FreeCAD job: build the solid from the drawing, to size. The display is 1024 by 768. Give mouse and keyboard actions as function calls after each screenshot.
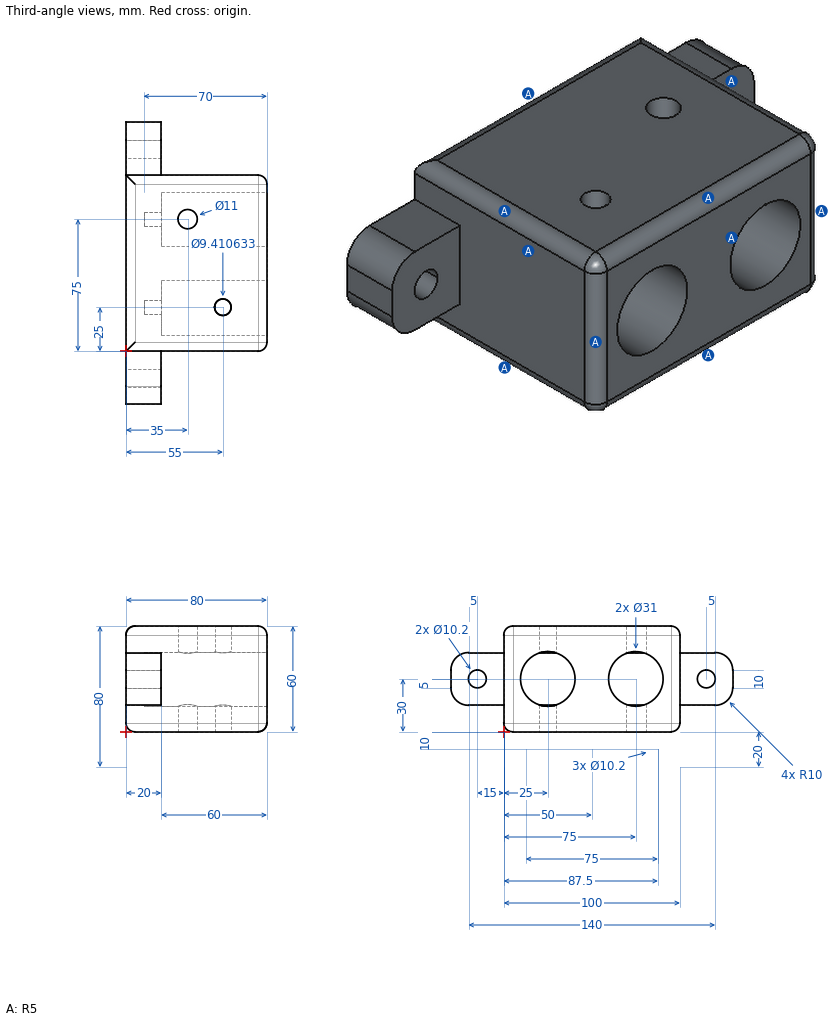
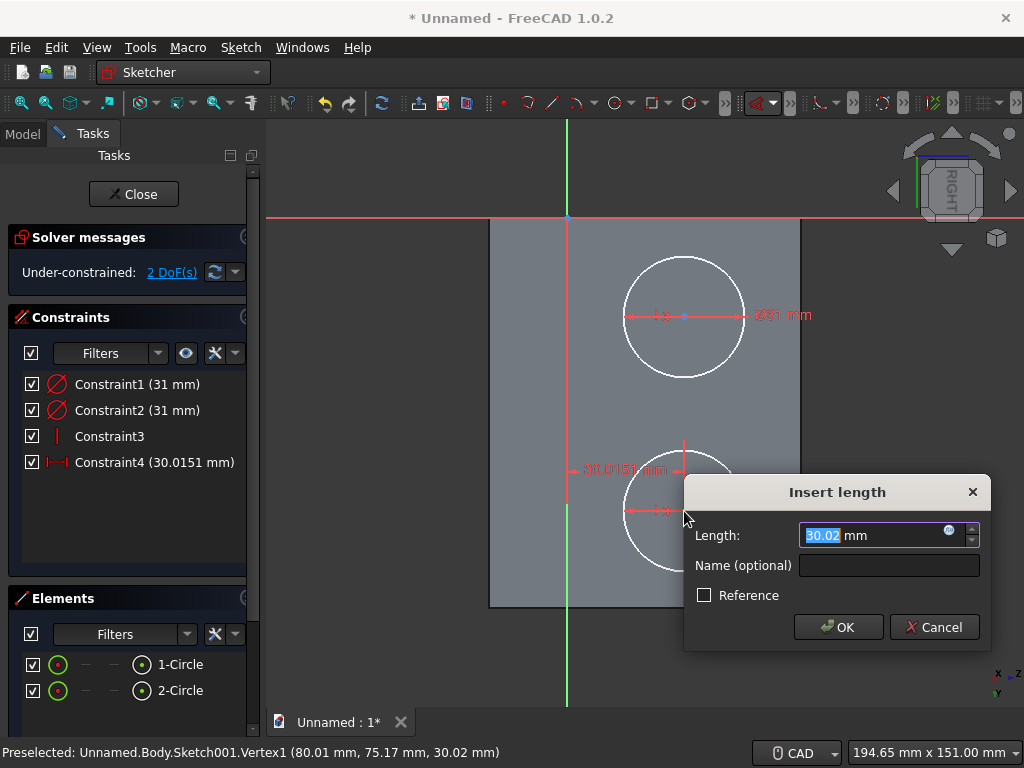
text(30)
key(Return)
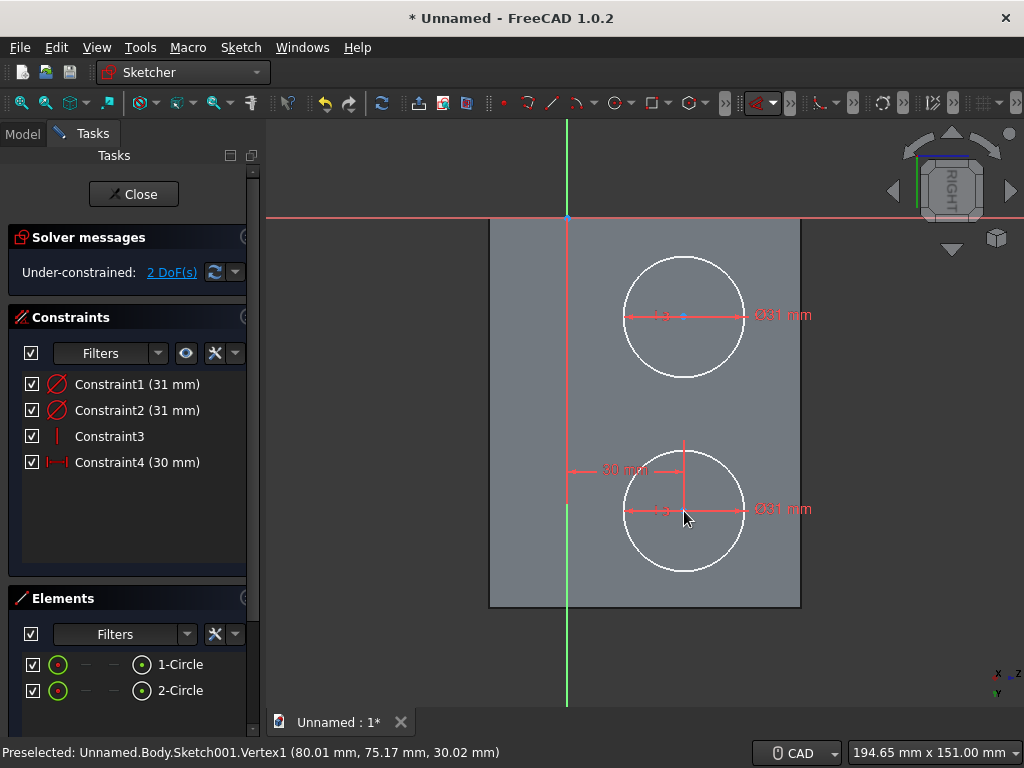
click(684, 511)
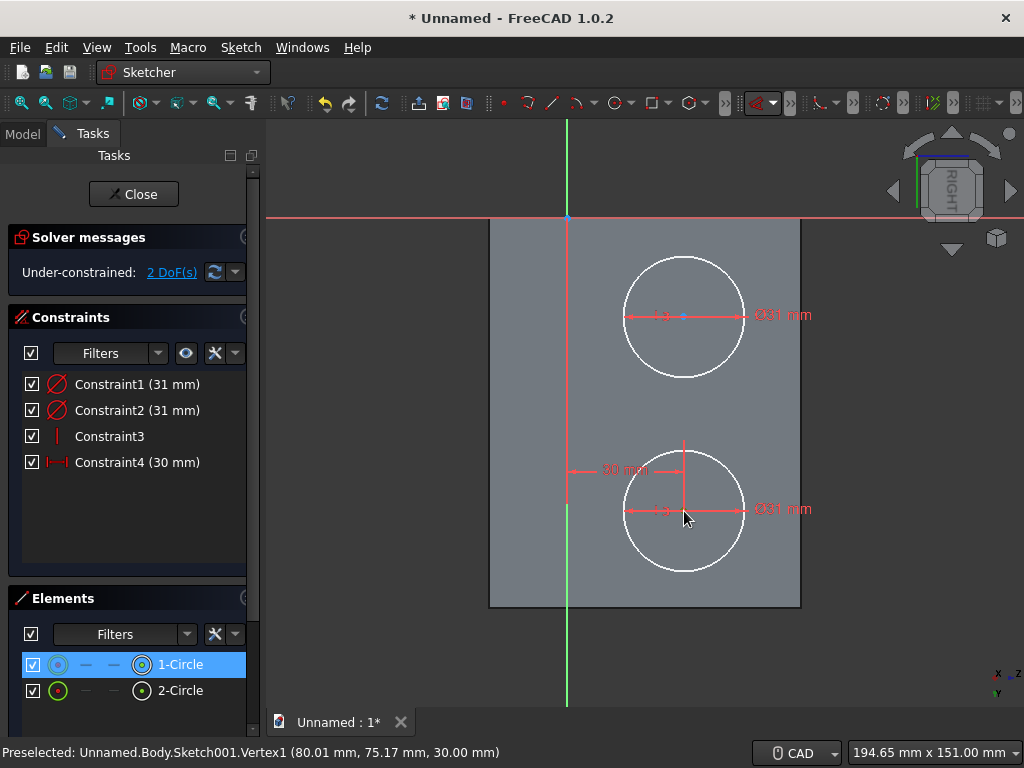
key(i)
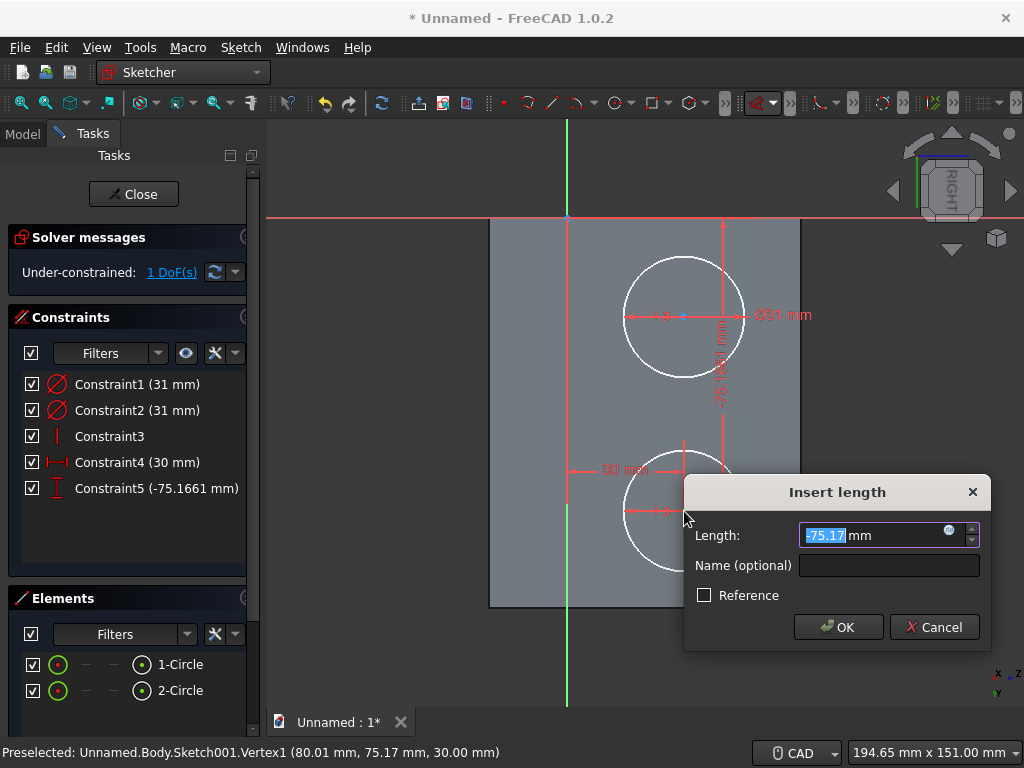
text(-75)
key(Return)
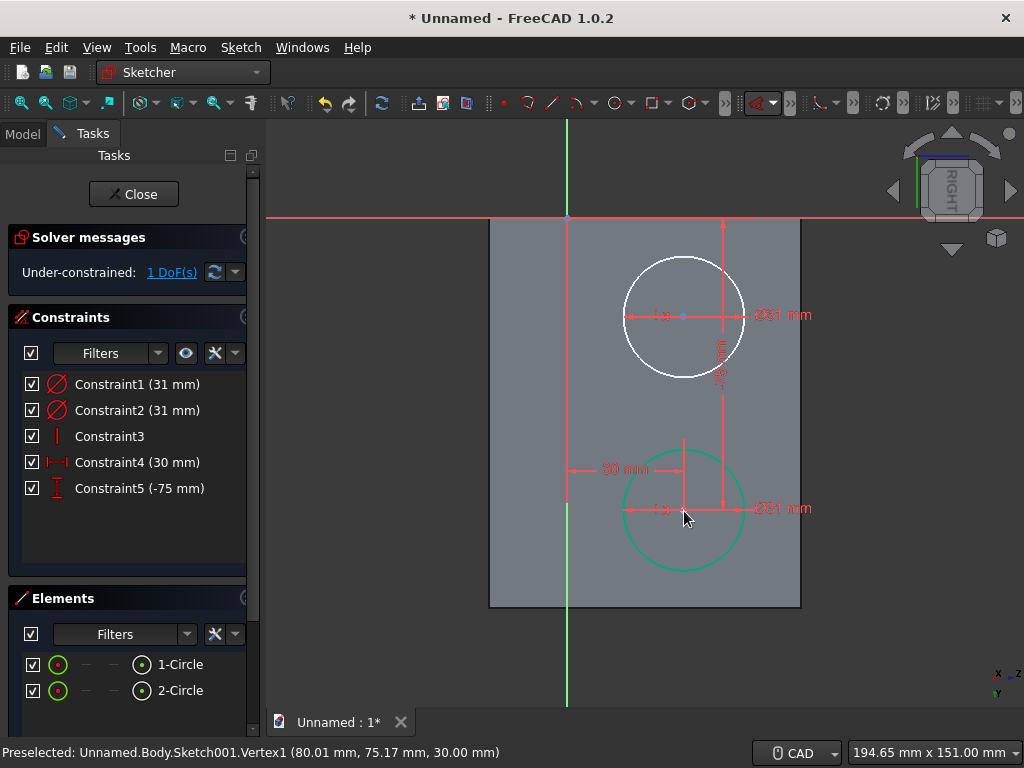
click(684, 317)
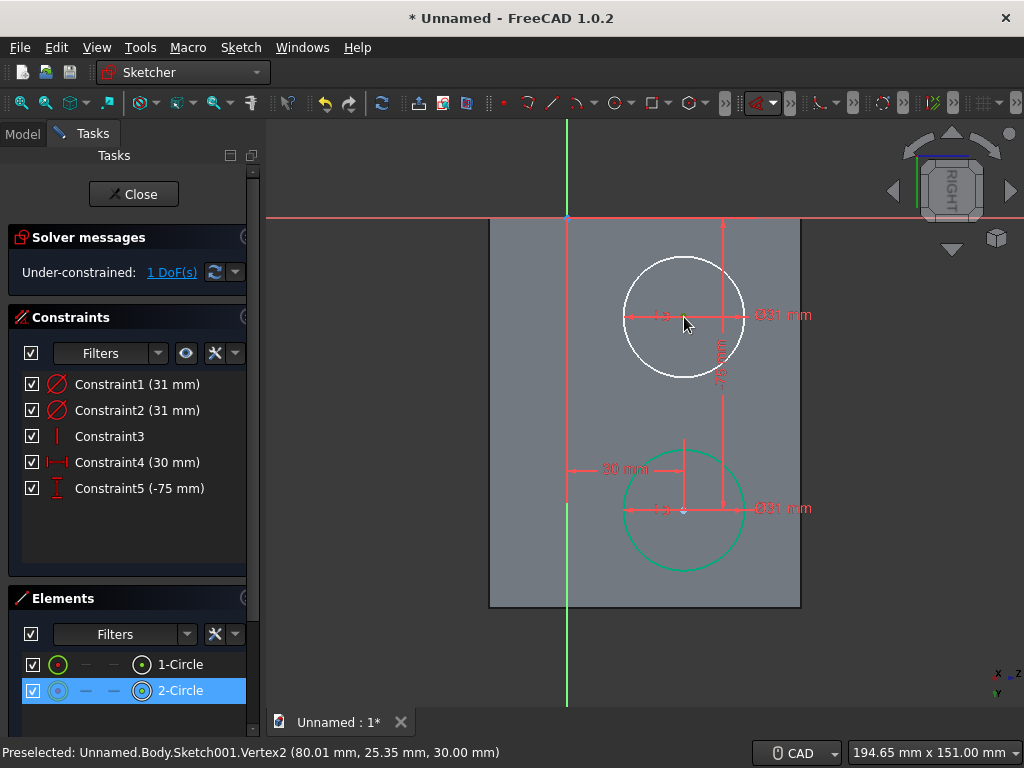
key(i)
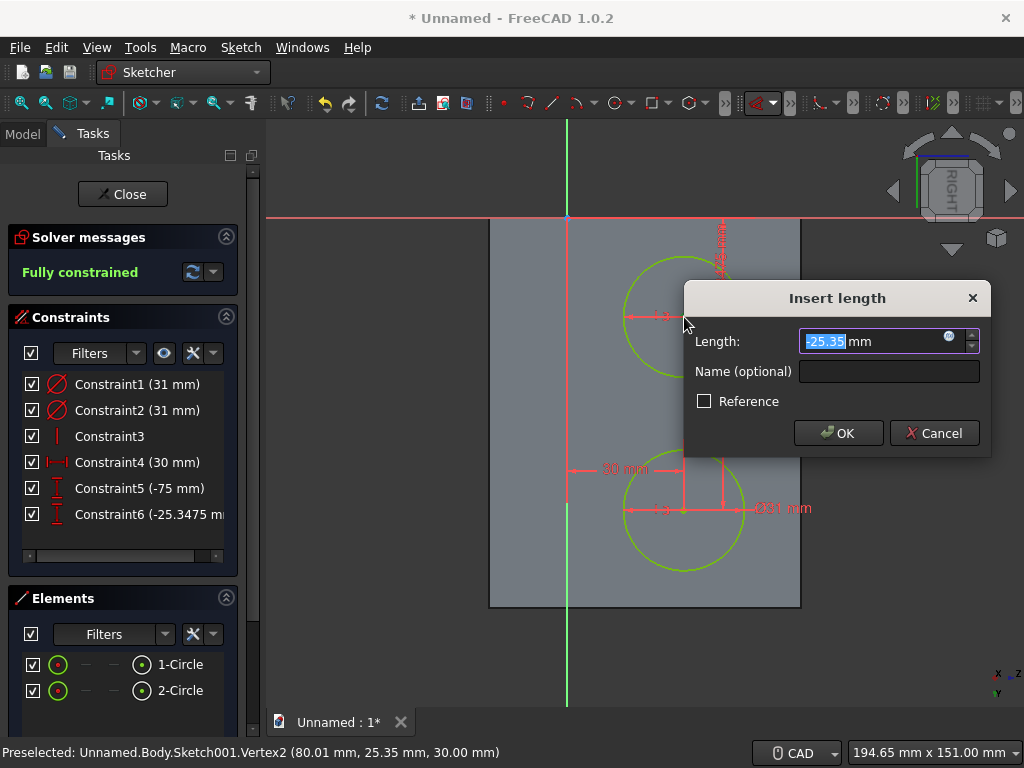
text(-25)
key(Return)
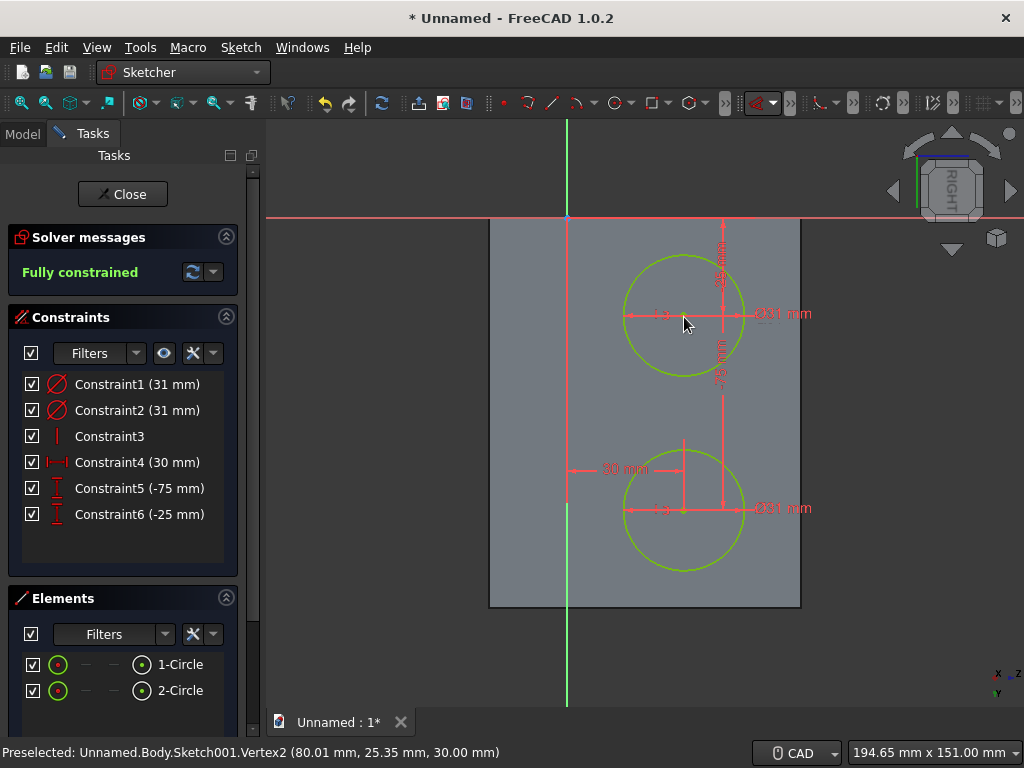
click(123, 194)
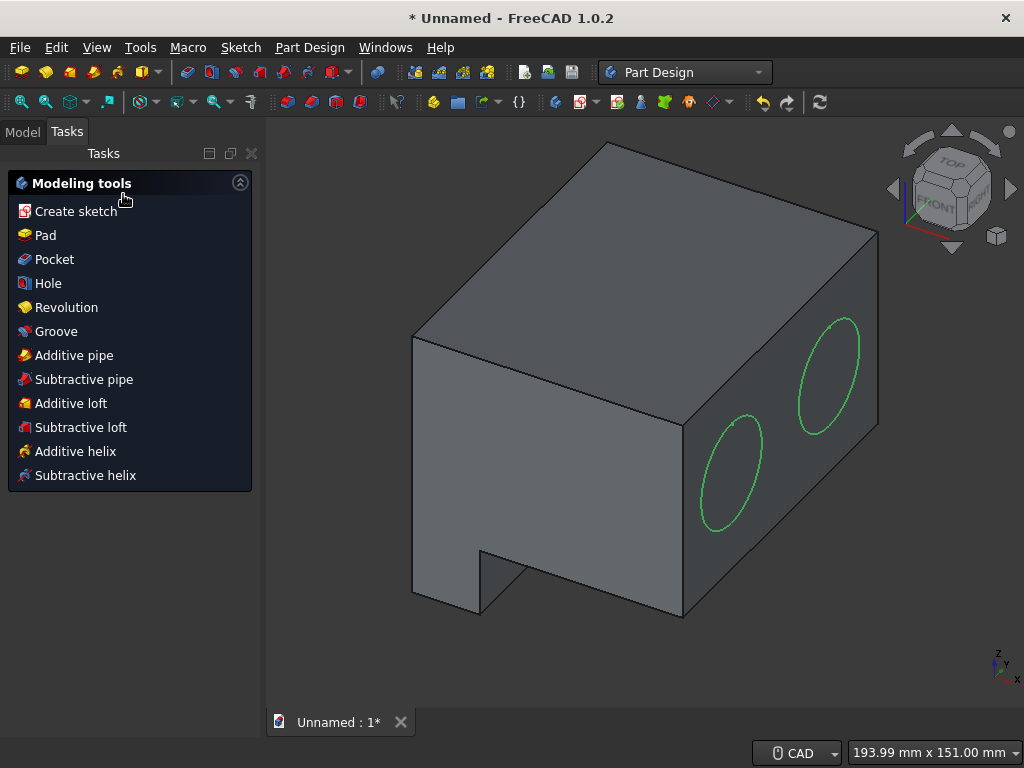
click(188, 72)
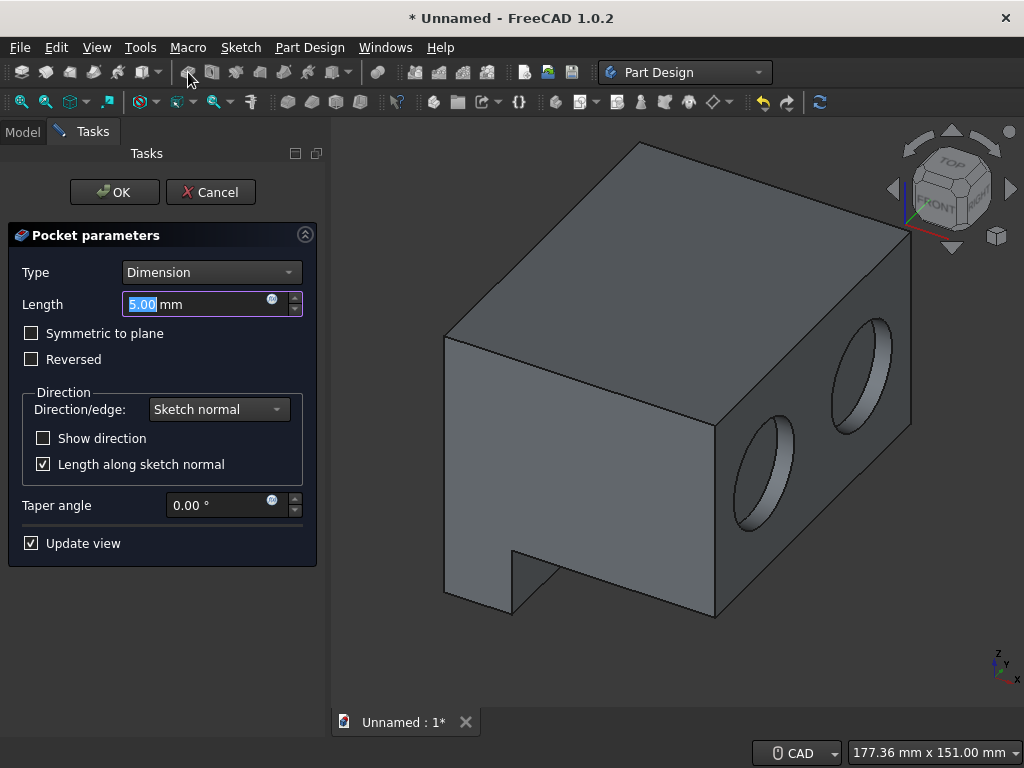
text(70)
key(Tab)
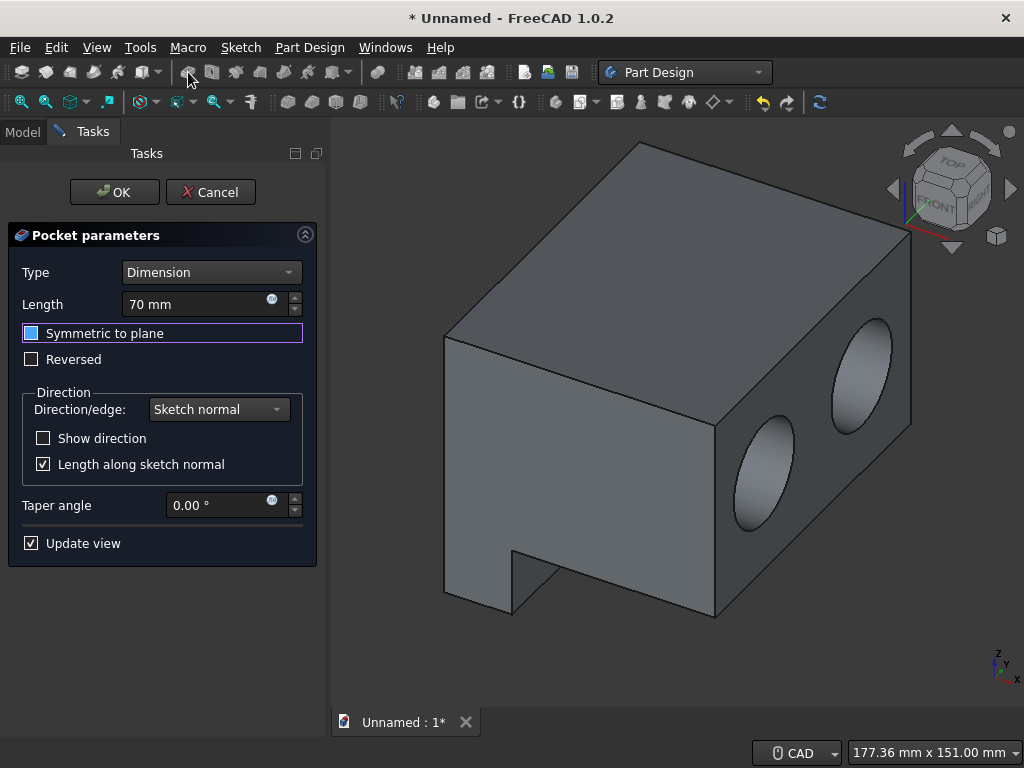
click(115, 192)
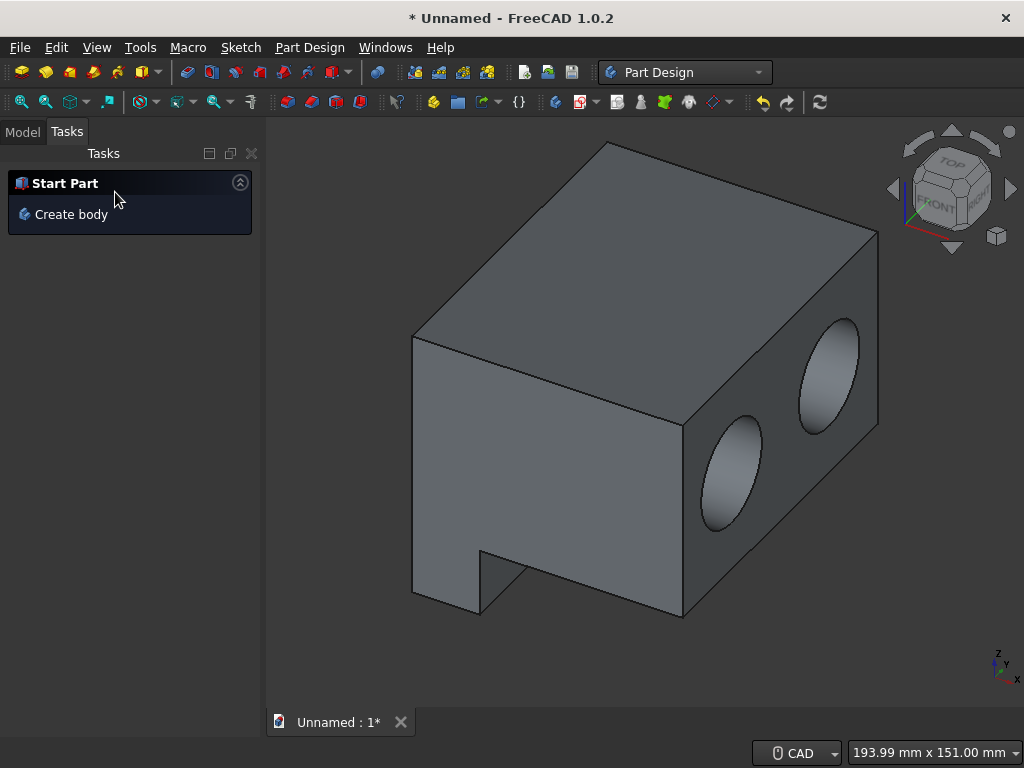
key(0)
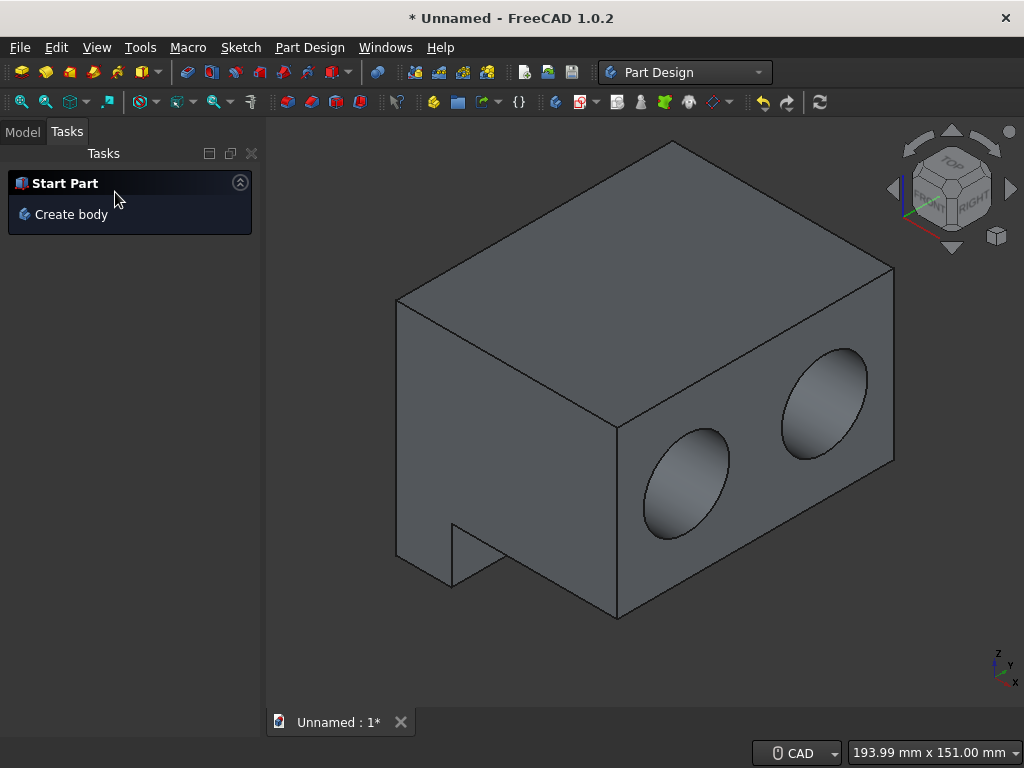
key(3)